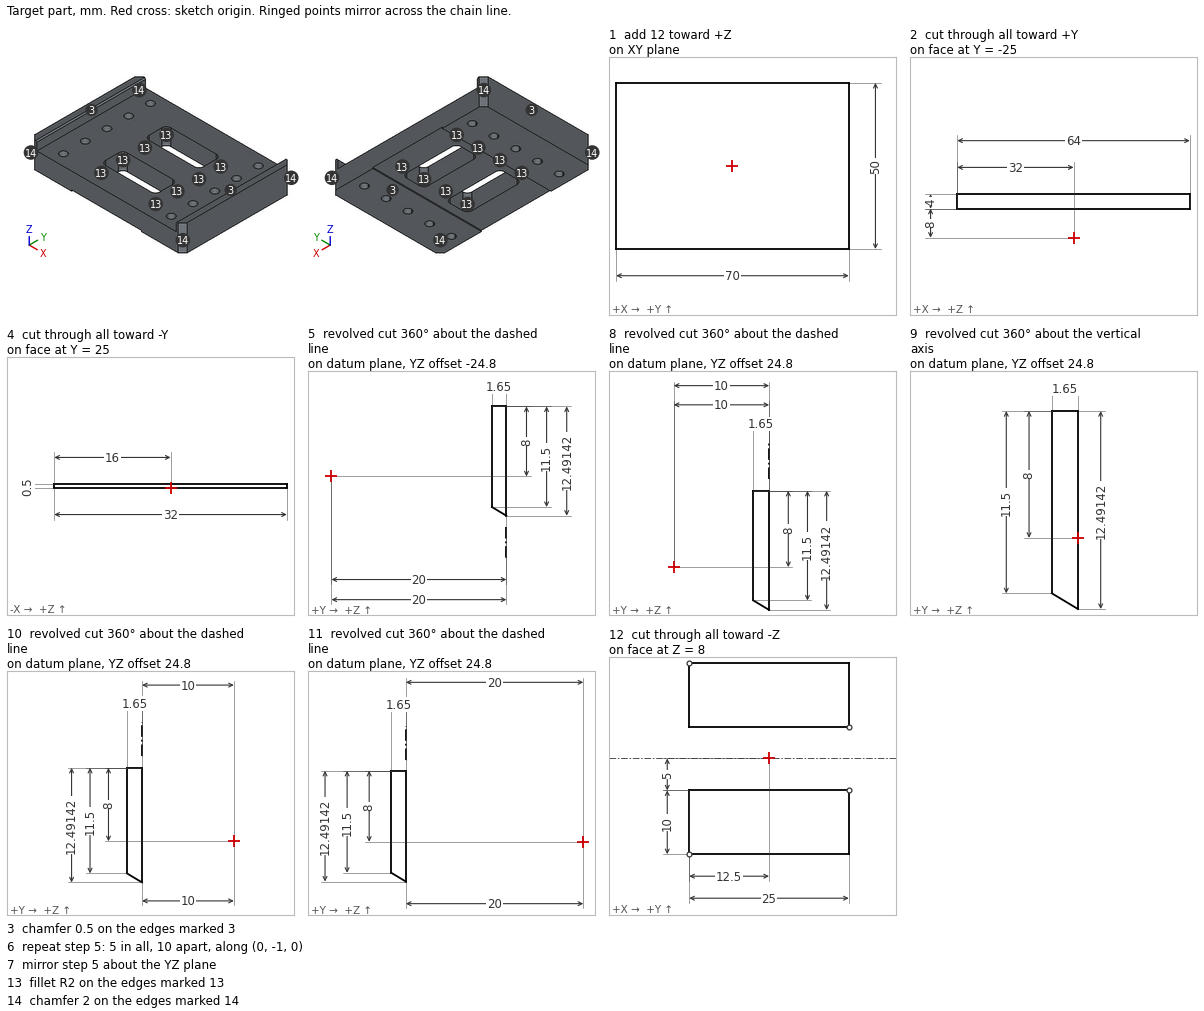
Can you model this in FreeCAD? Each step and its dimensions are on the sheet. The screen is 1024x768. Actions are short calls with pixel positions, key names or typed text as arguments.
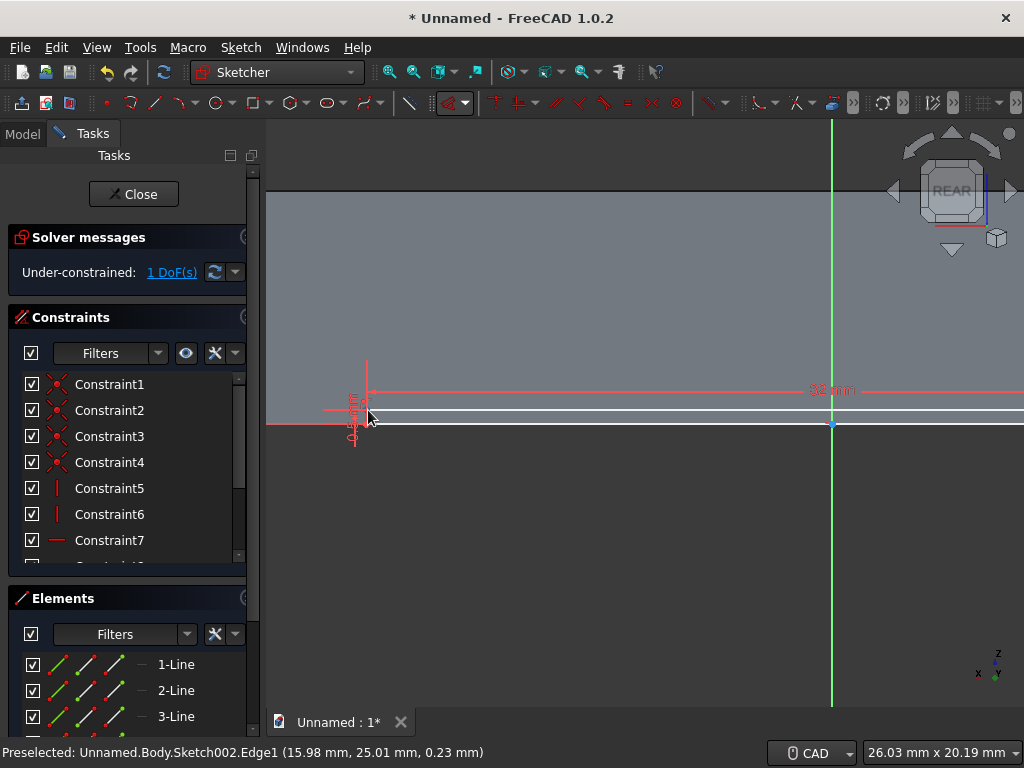
click(367, 410)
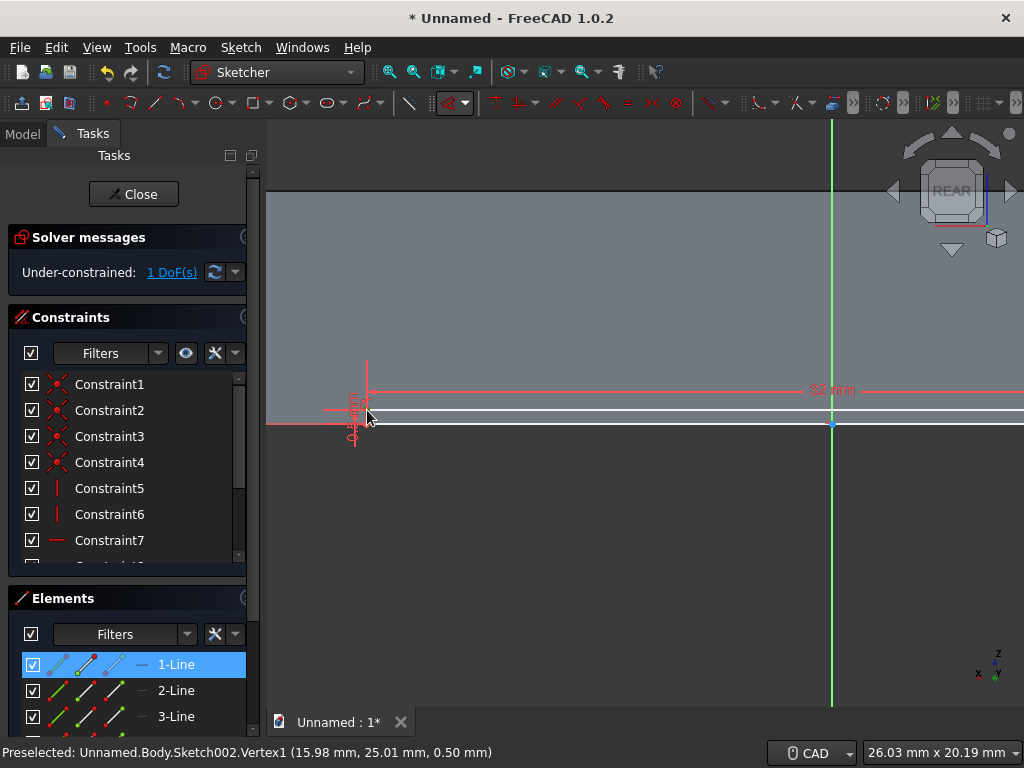
key(l)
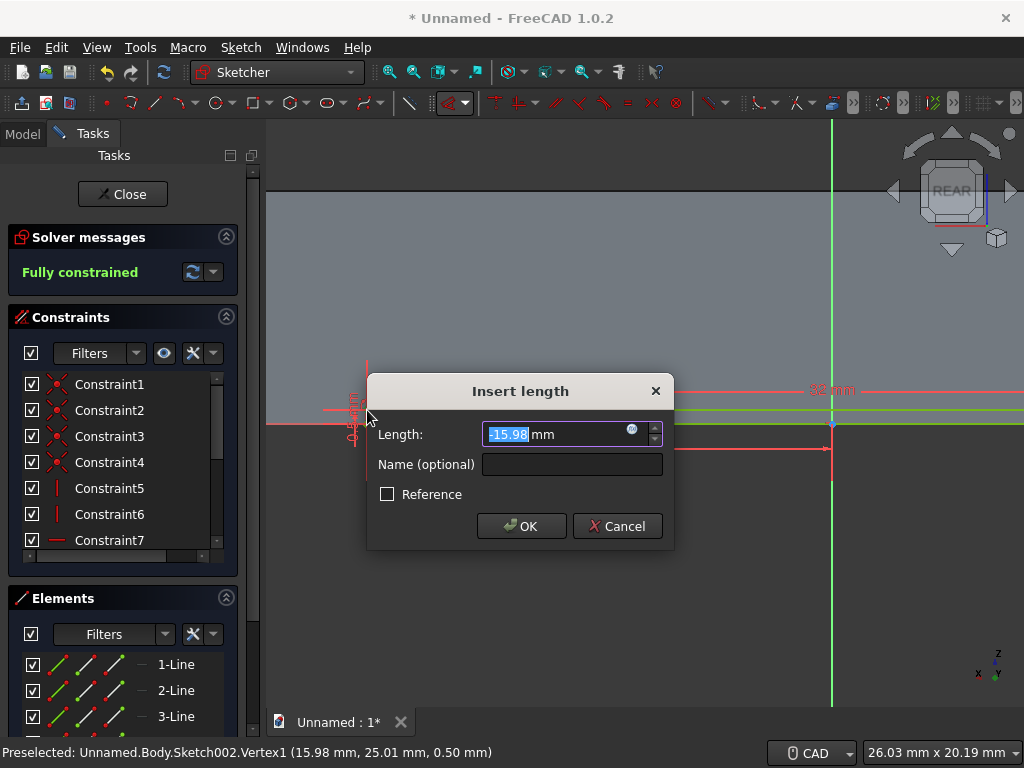
text(-16)
key(Return)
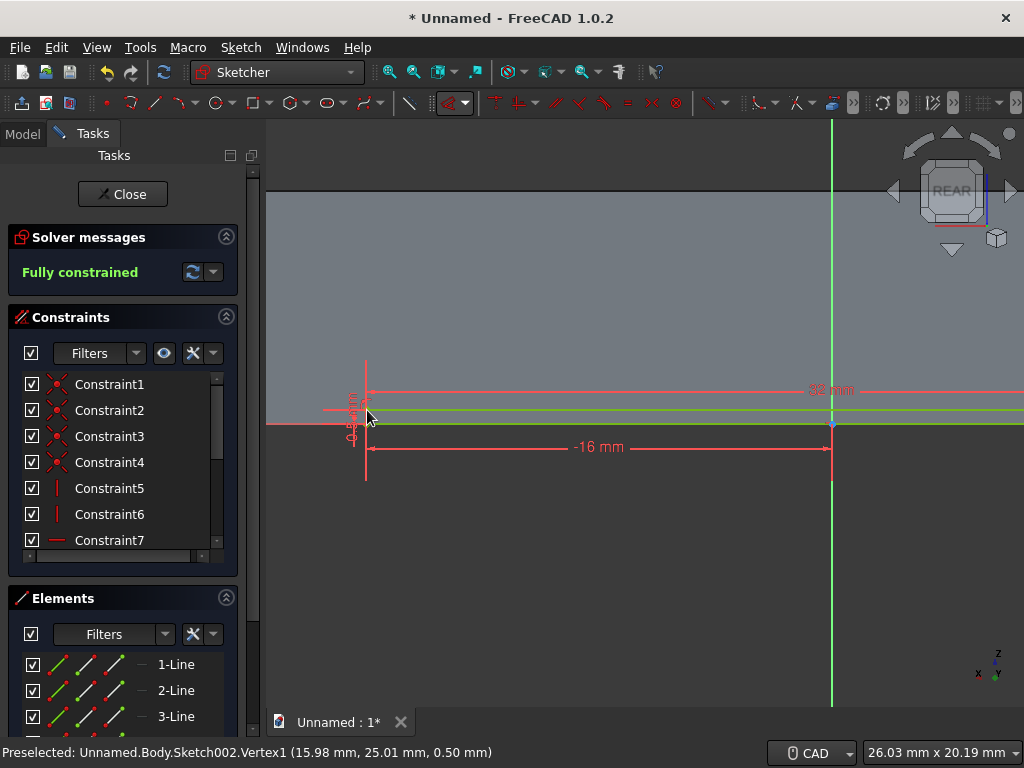
click(123, 194)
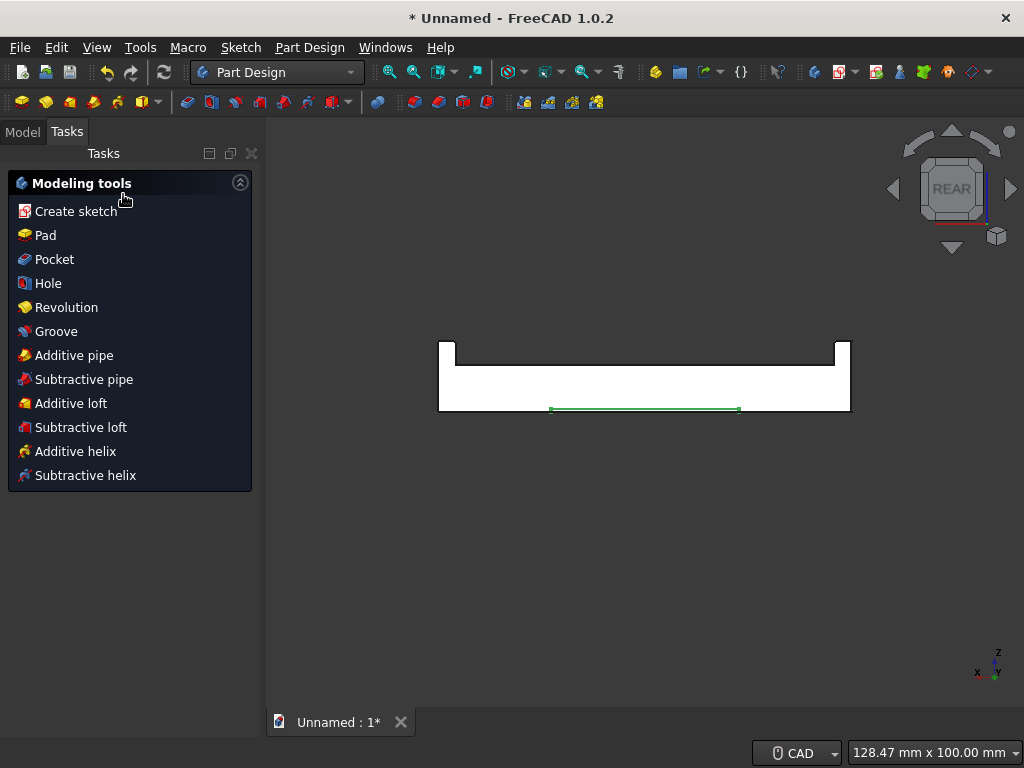
click(188, 102)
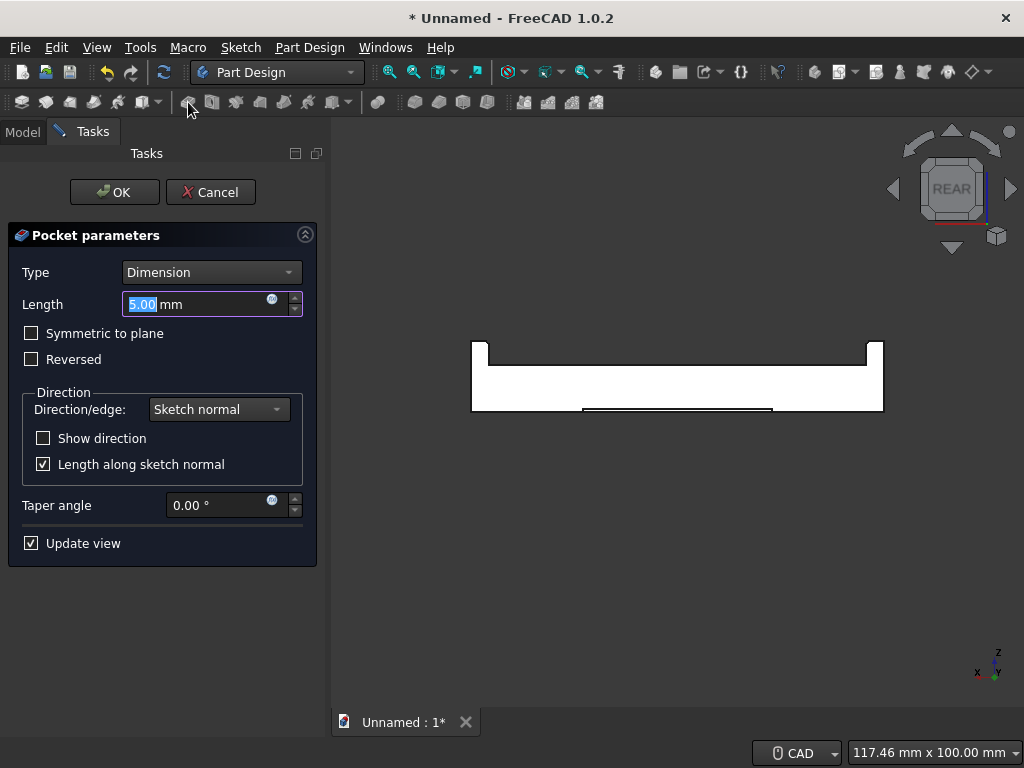
click(212, 272)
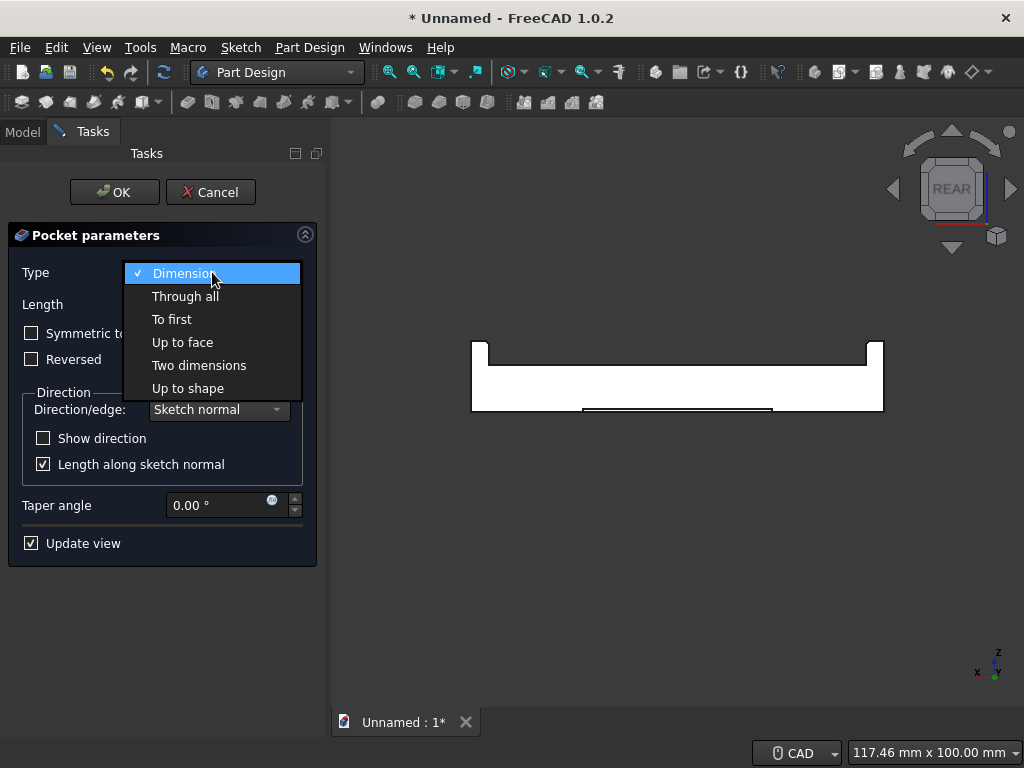
click(212, 296)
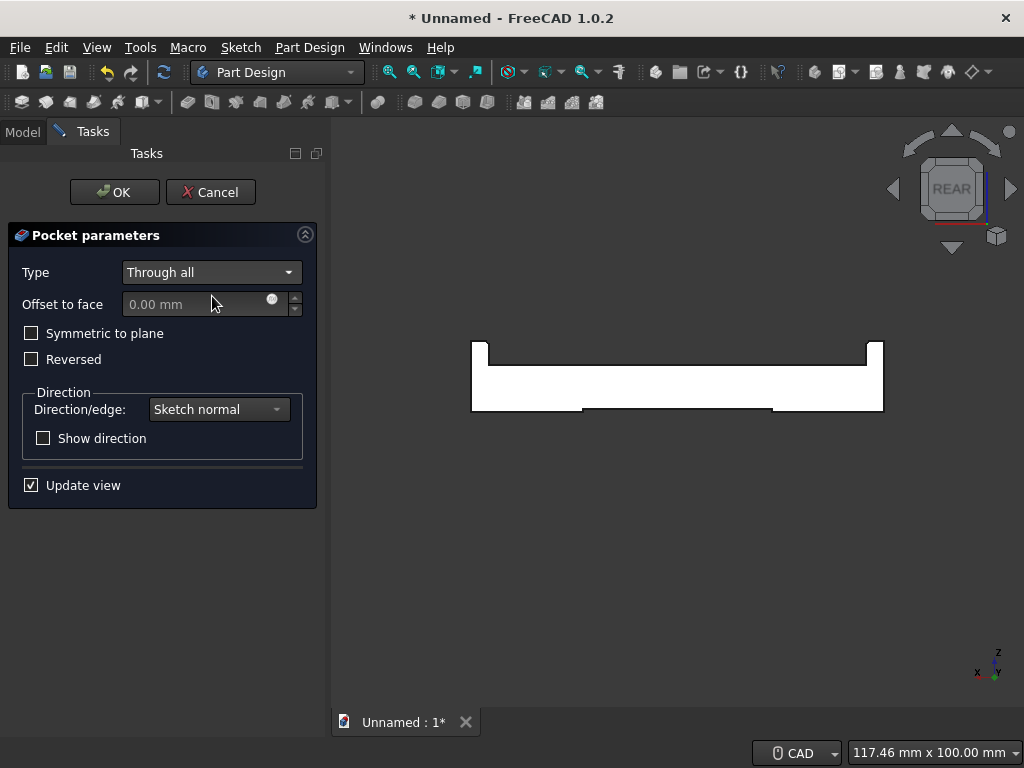
click(115, 192)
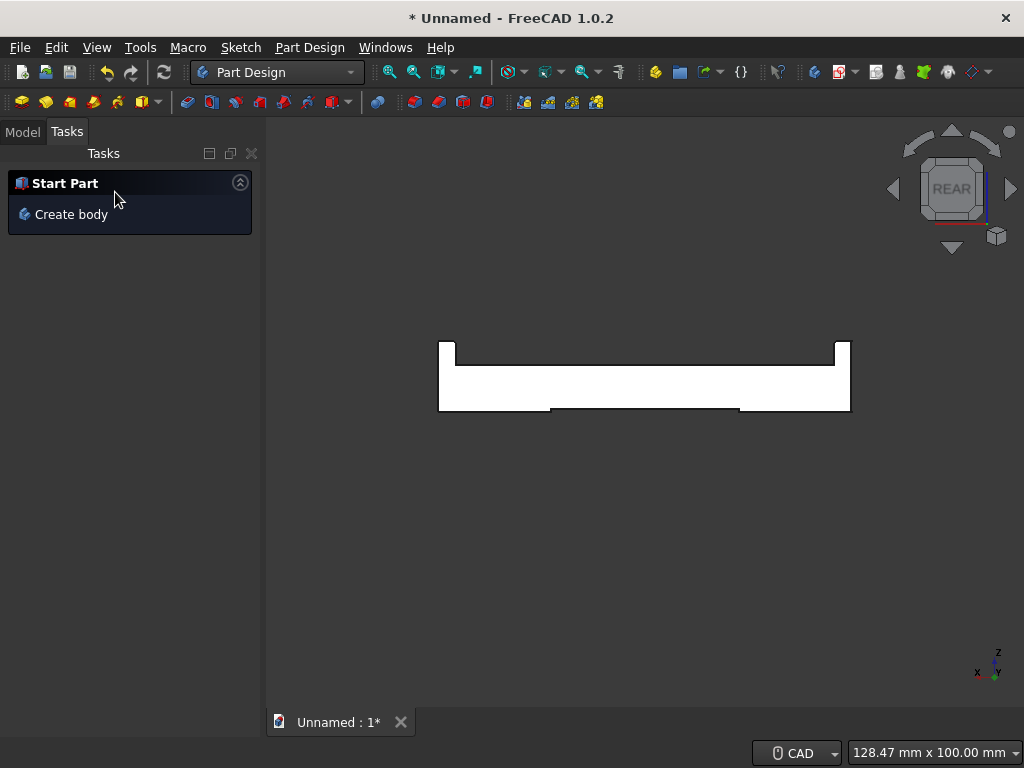
click(23, 131)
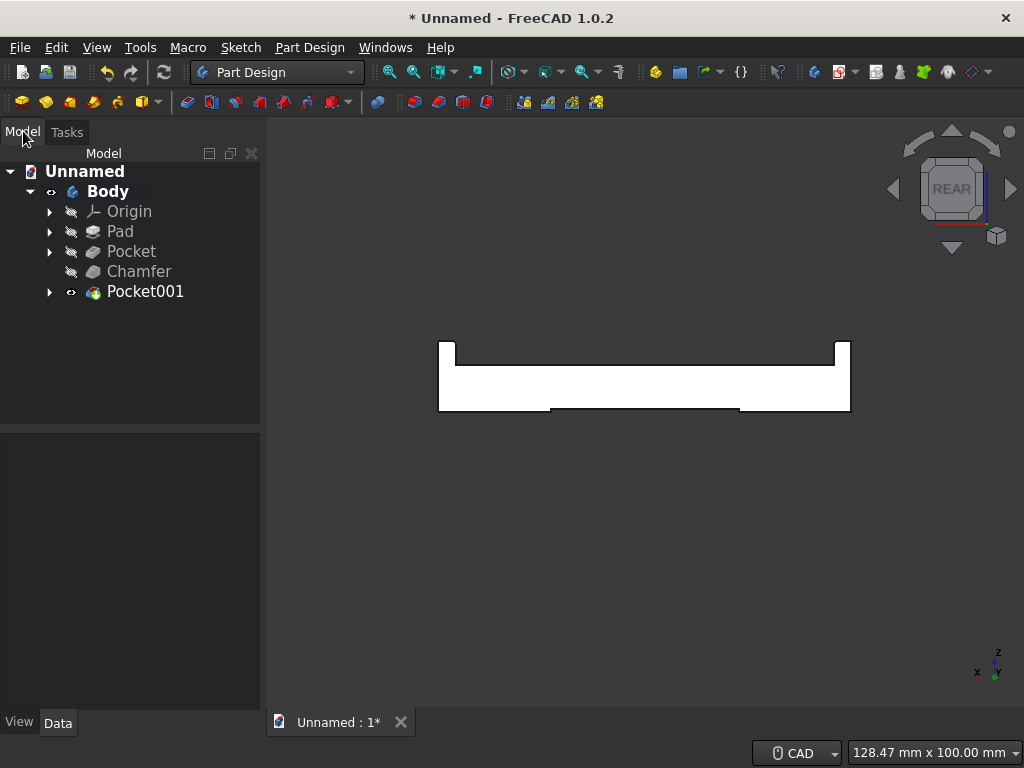
click(50, 212)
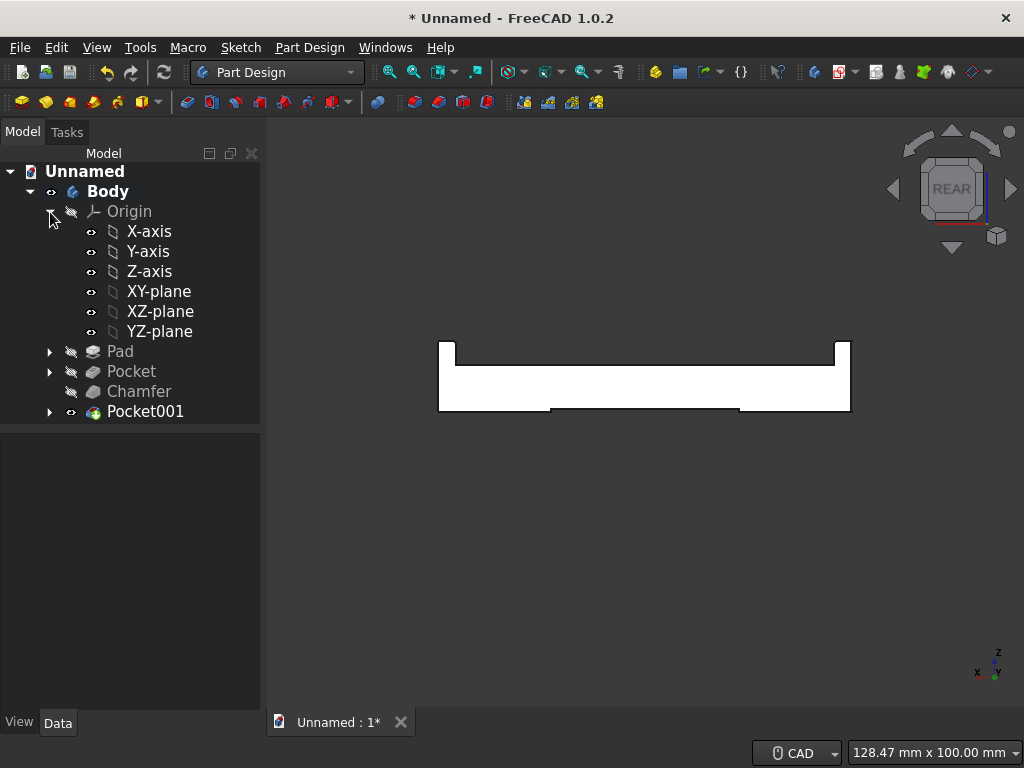
click(136, 332)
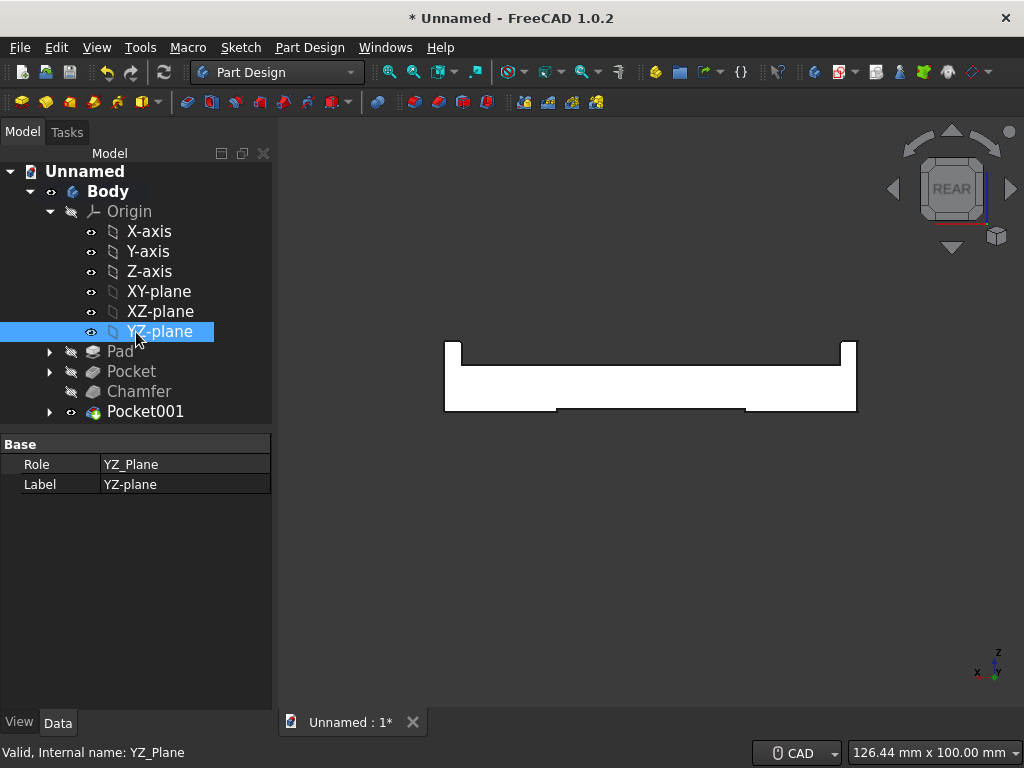
click(972, 72)